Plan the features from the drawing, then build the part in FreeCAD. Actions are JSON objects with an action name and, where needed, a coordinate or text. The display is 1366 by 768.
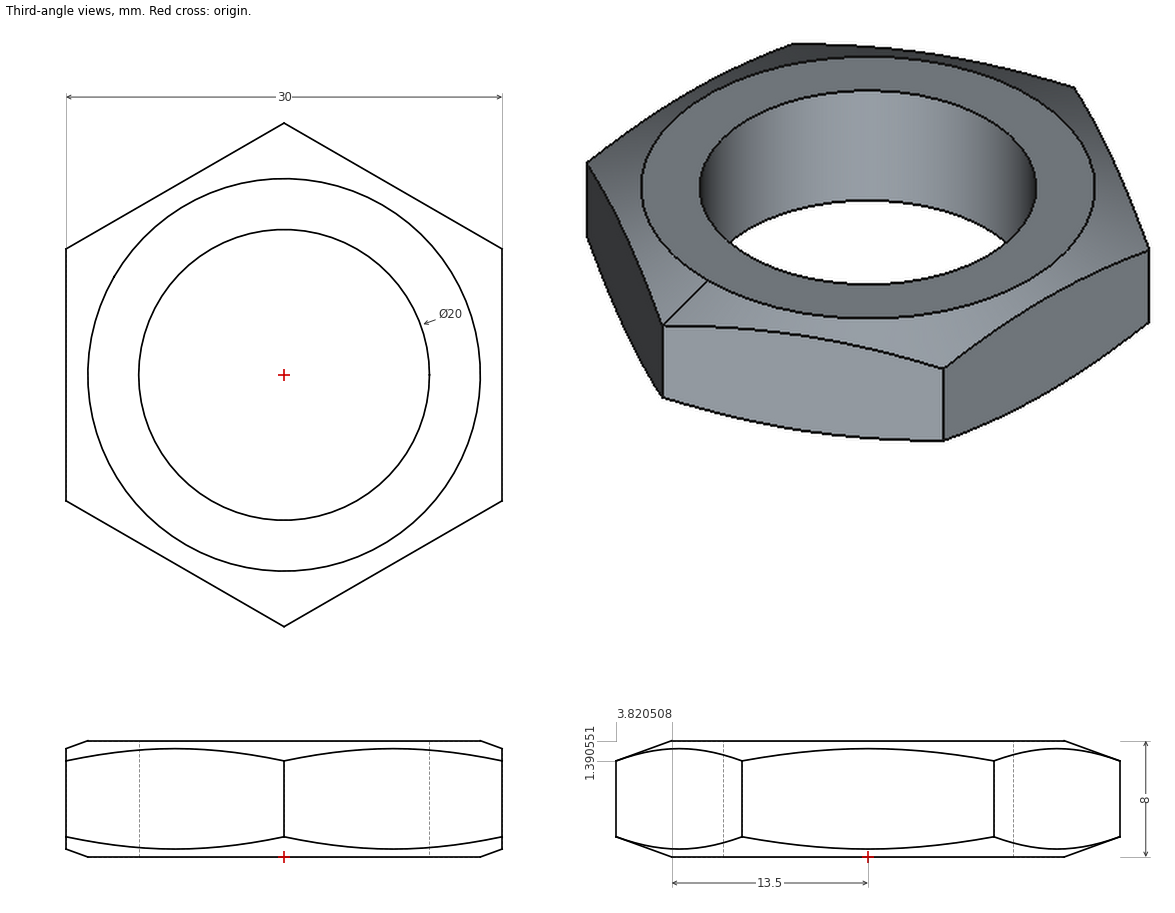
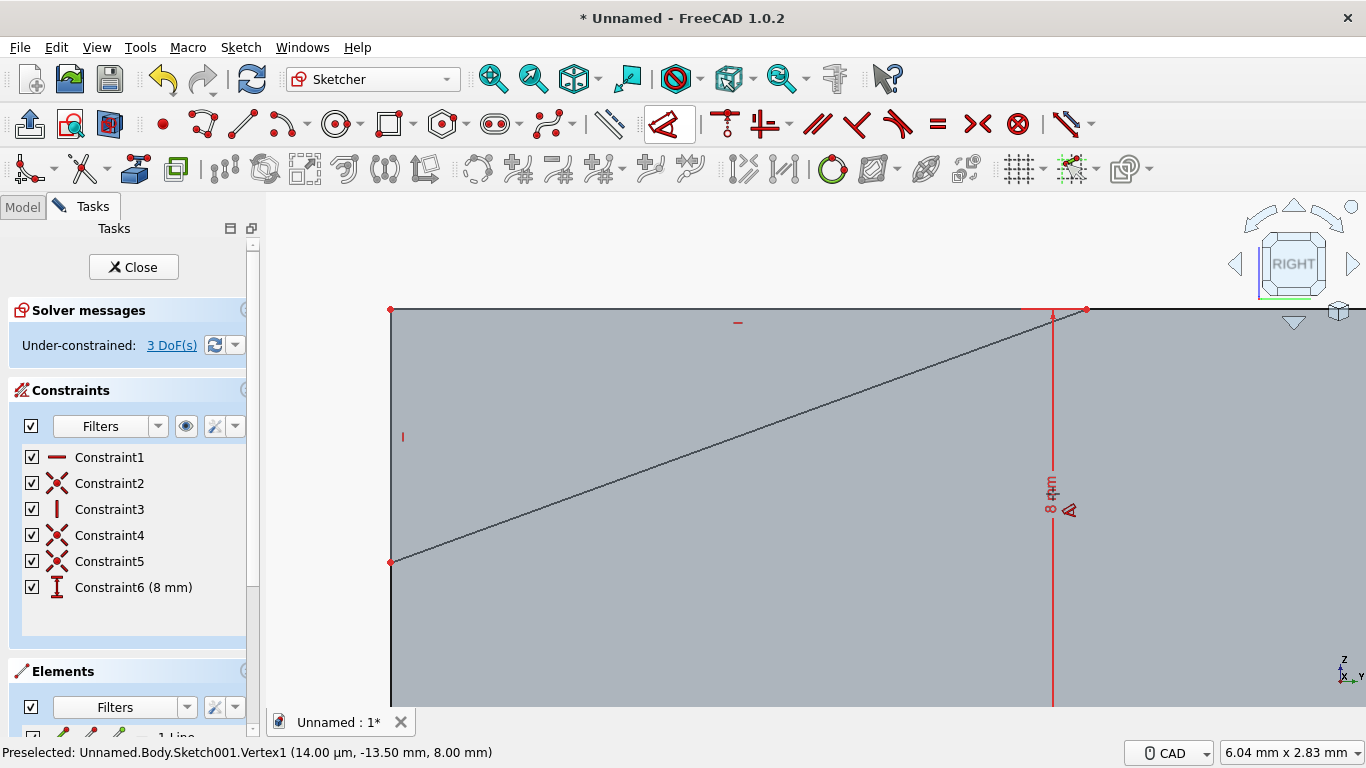
{"action": "left_click", "coordinate": [1087, 309]}
{"action": "left_click", "coordinate": [1144, 275]}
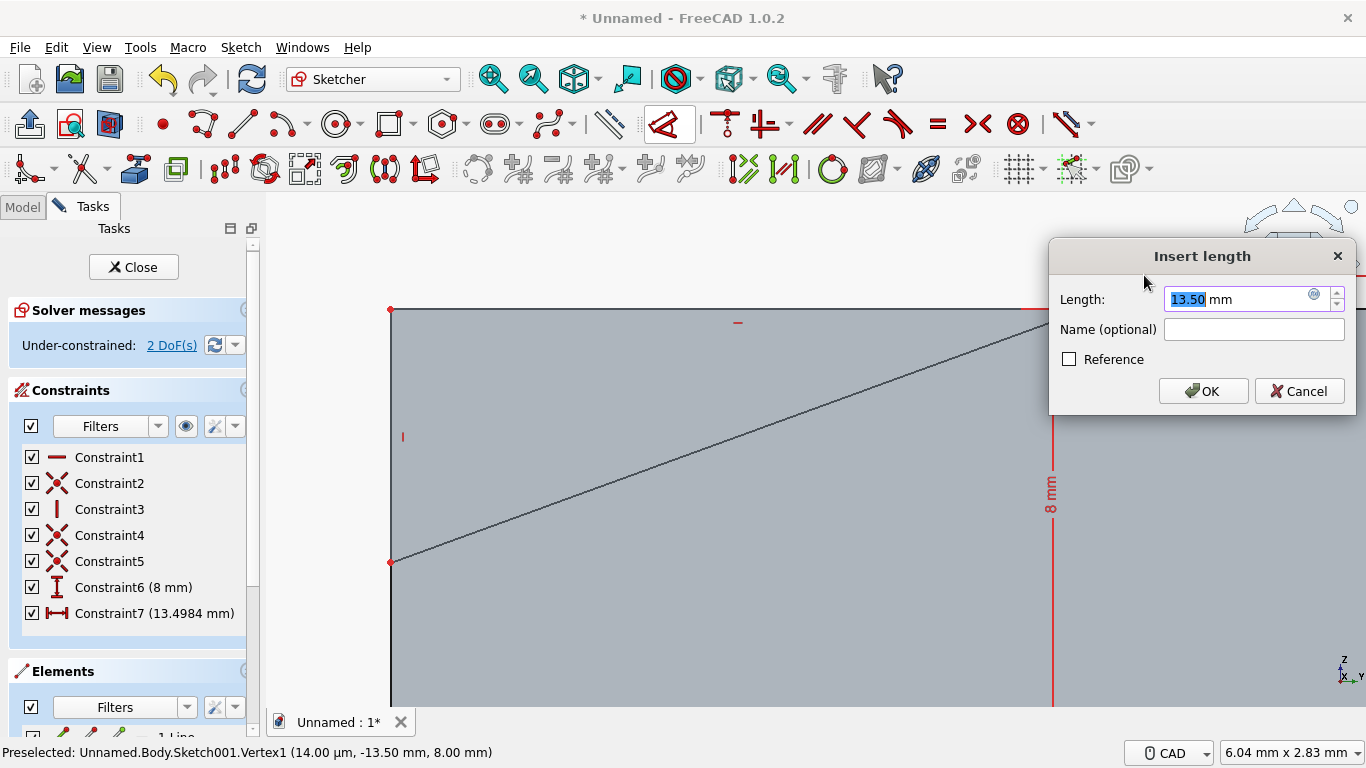
{"action": "type", "text": "13.5"}
{"action": "key", "text": "Return"}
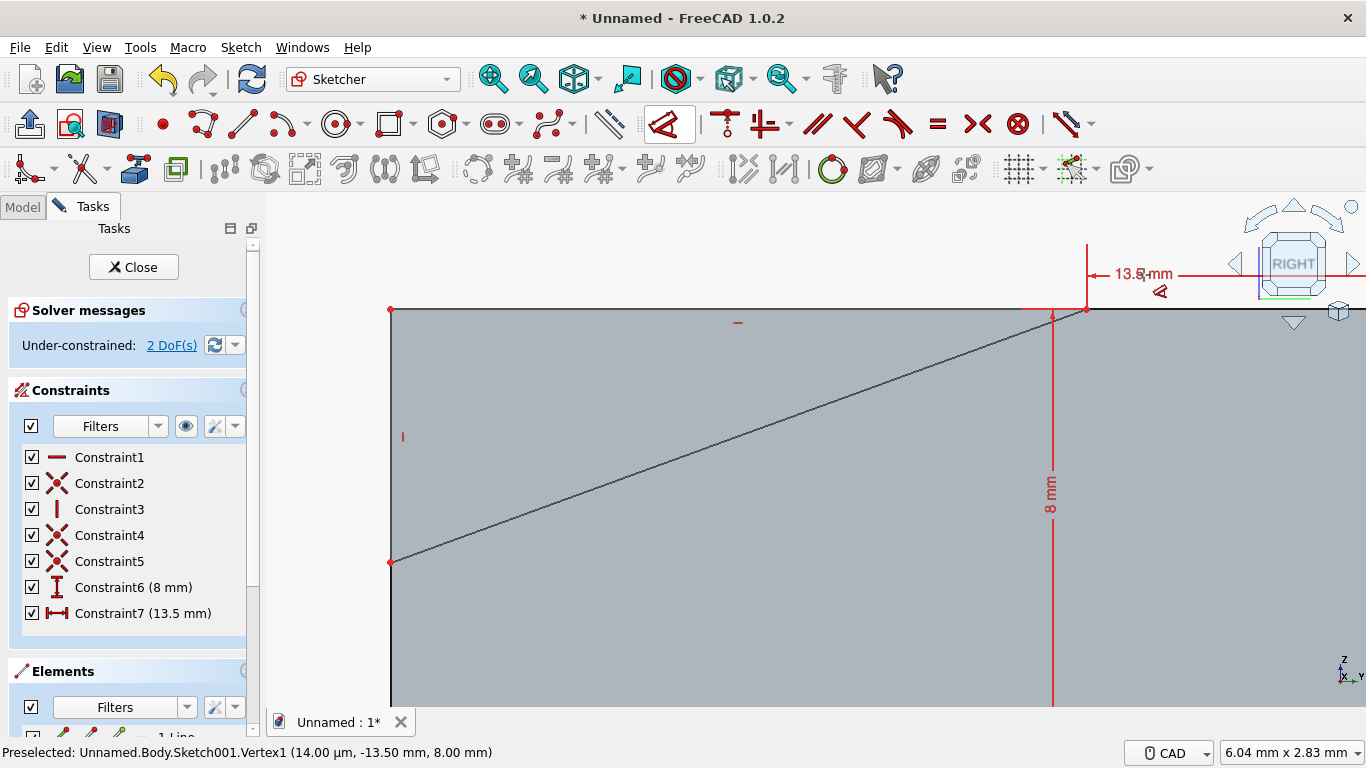
{"action": "left_click", "coordinate": [878, 309]}
{"action": "left_click", "coordinate": [739, 275]}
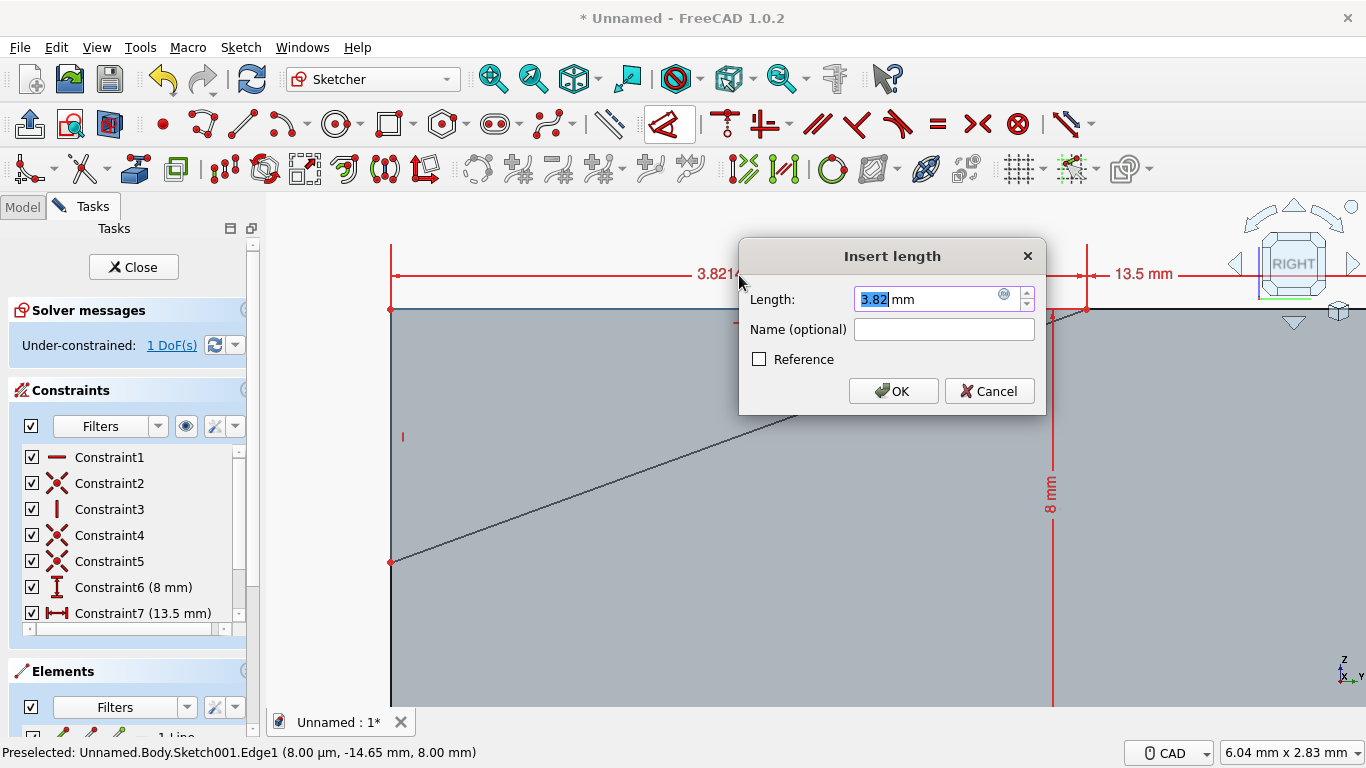
{"action": "type", "text": "3.820508"}
{"action": "key", "text": "Return"}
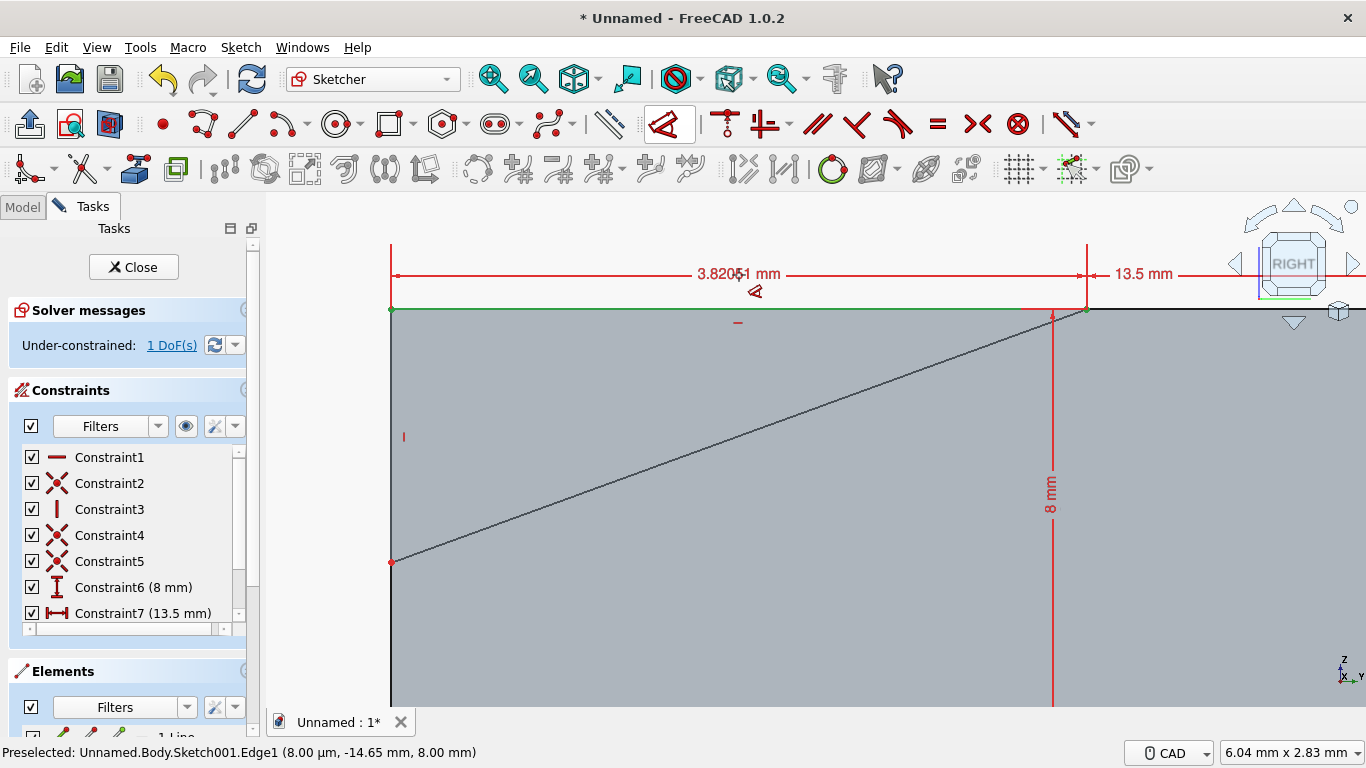
{"action": "left_click", "coordinate": [391, 385]}
{"action": "left_click", "coordinate": [357, 436]}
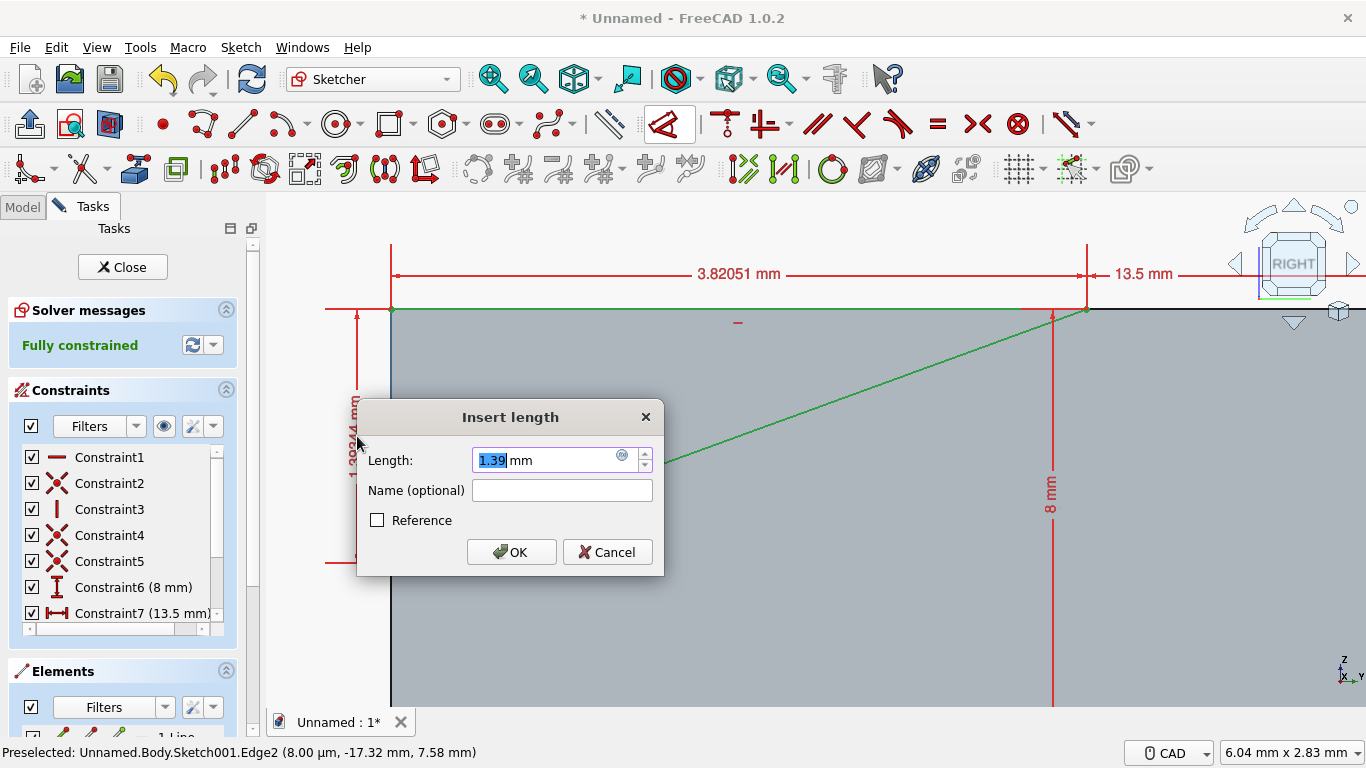
{"action": "type", "text": "1.390551"}
{"action": "key", "text": "Return"}
{"action": "key", "text": "Escape"}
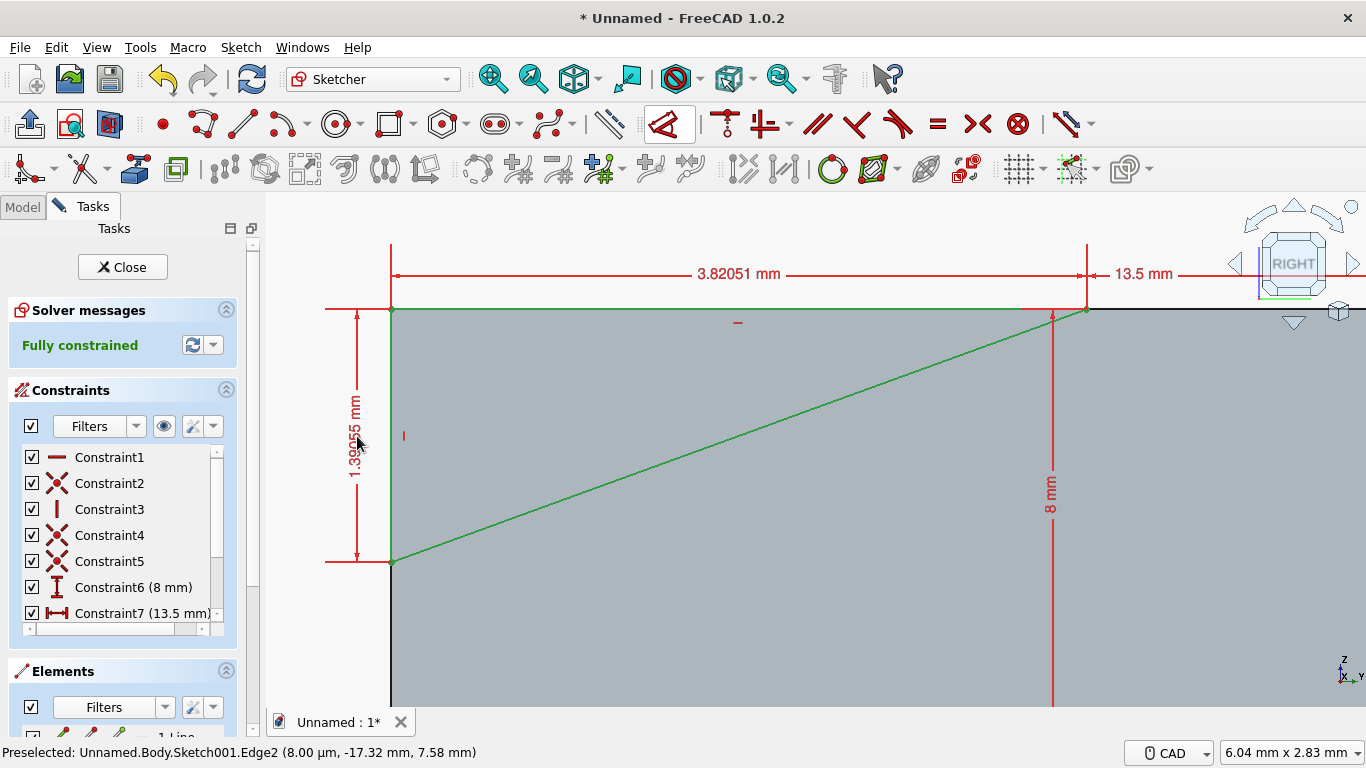
{"action": "left_click", "coordinate": [123, 267]}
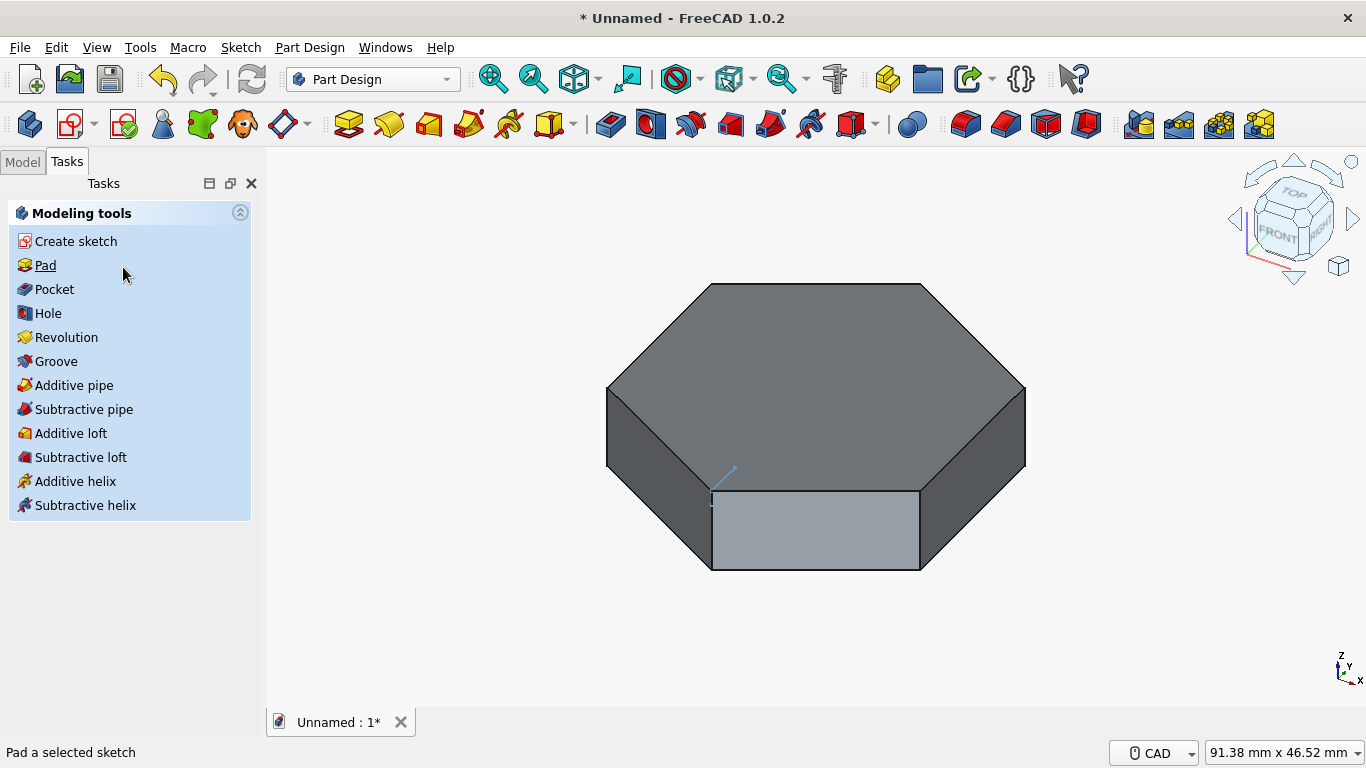
{"action": "left_click", "coordinate": [692, 124]}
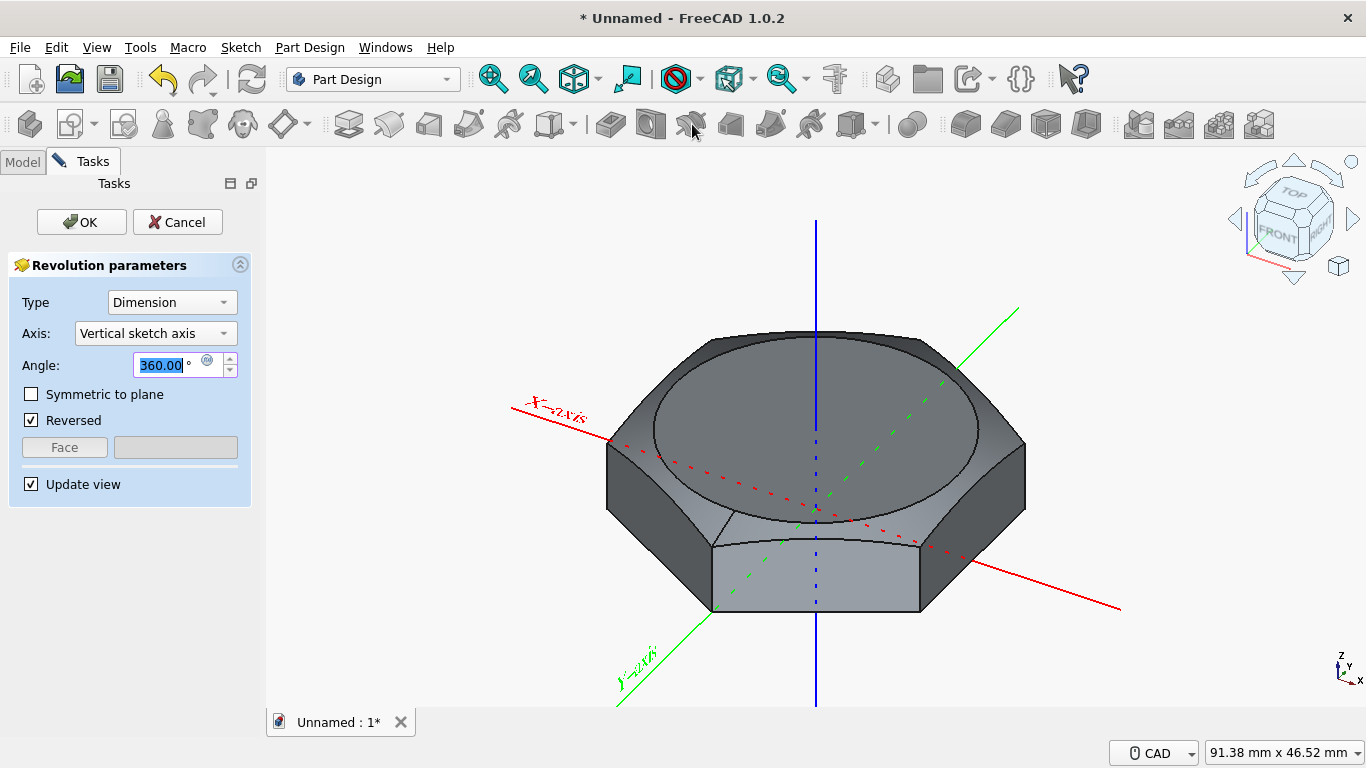
{"action": "left_click", "coordinate": [82, 222]}